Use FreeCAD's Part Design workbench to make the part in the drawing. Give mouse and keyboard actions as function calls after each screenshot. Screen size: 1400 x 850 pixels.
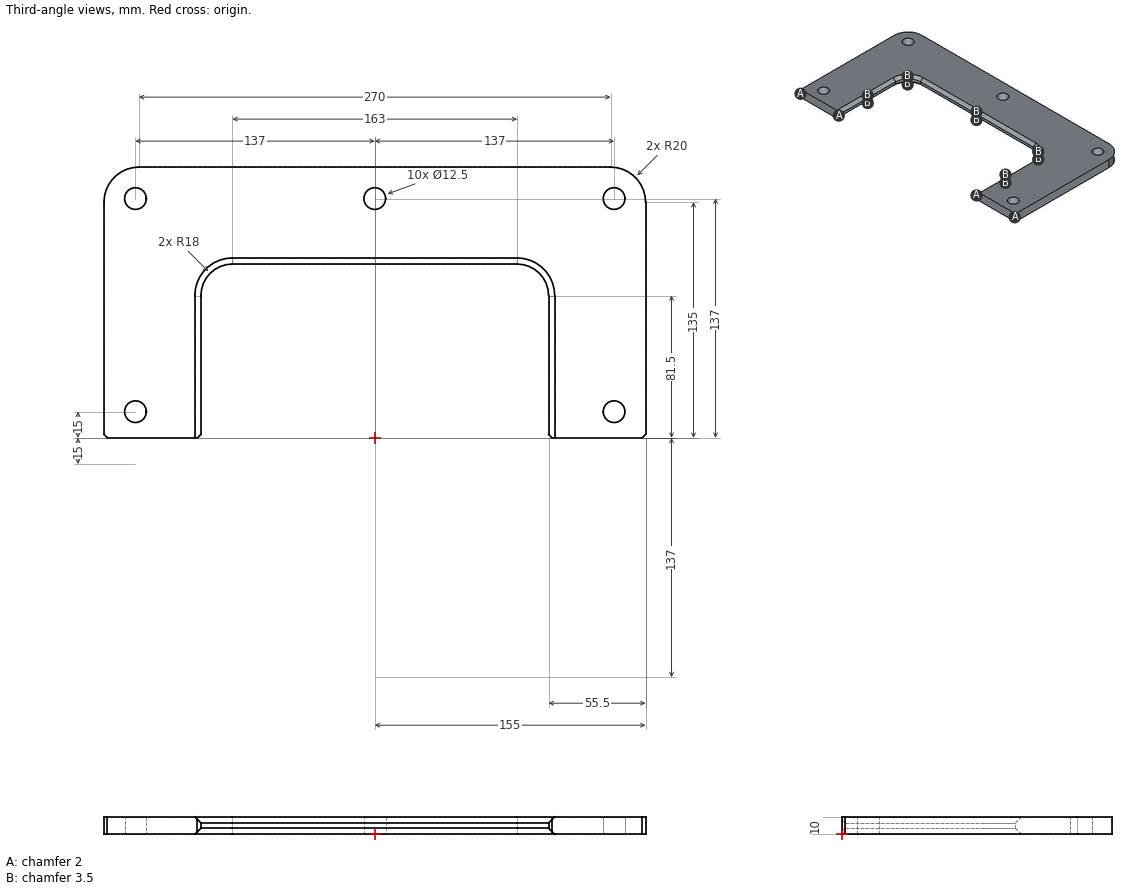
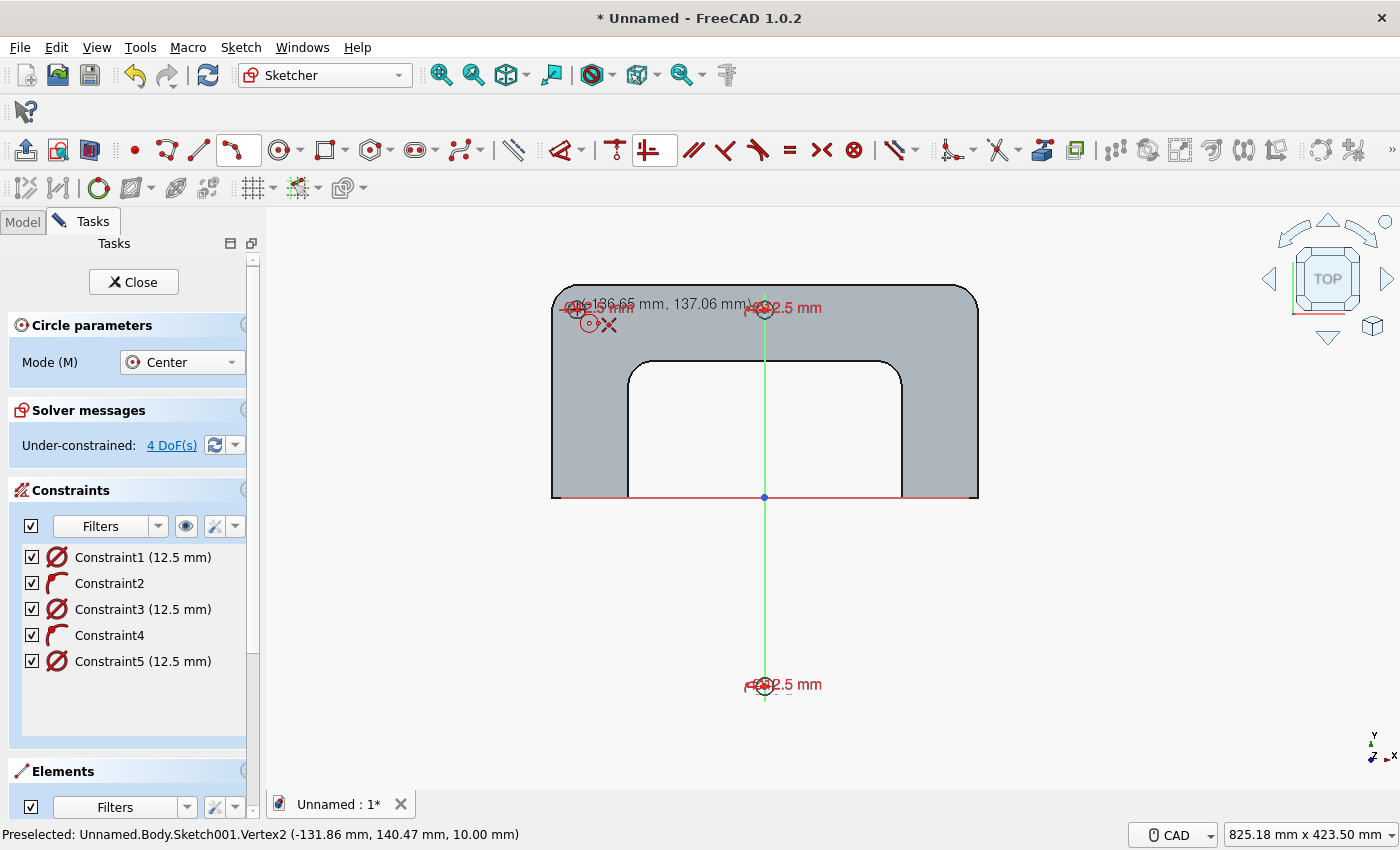
scroll(953, 310, up, 5)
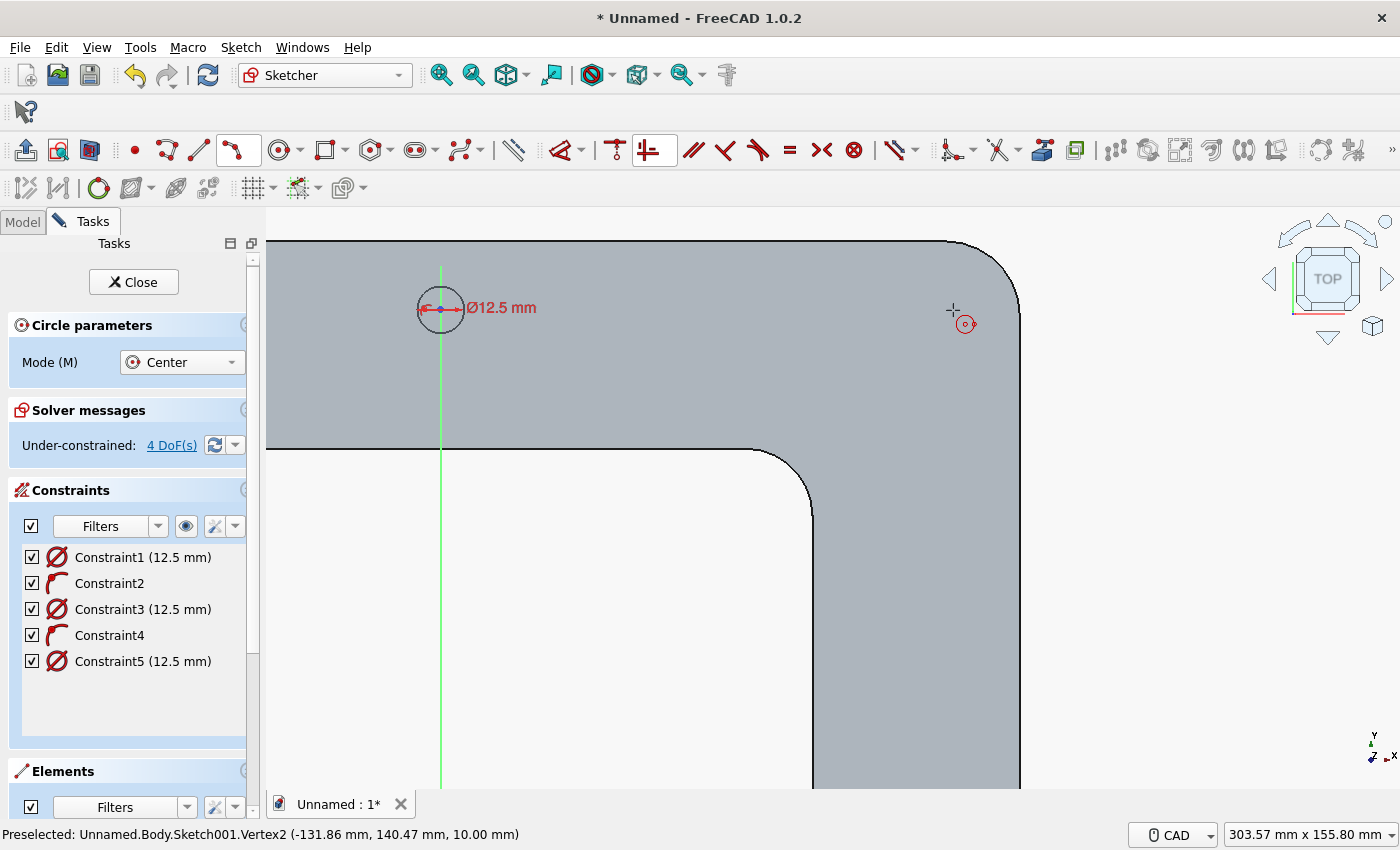
click(953, 309)
move(969, 292)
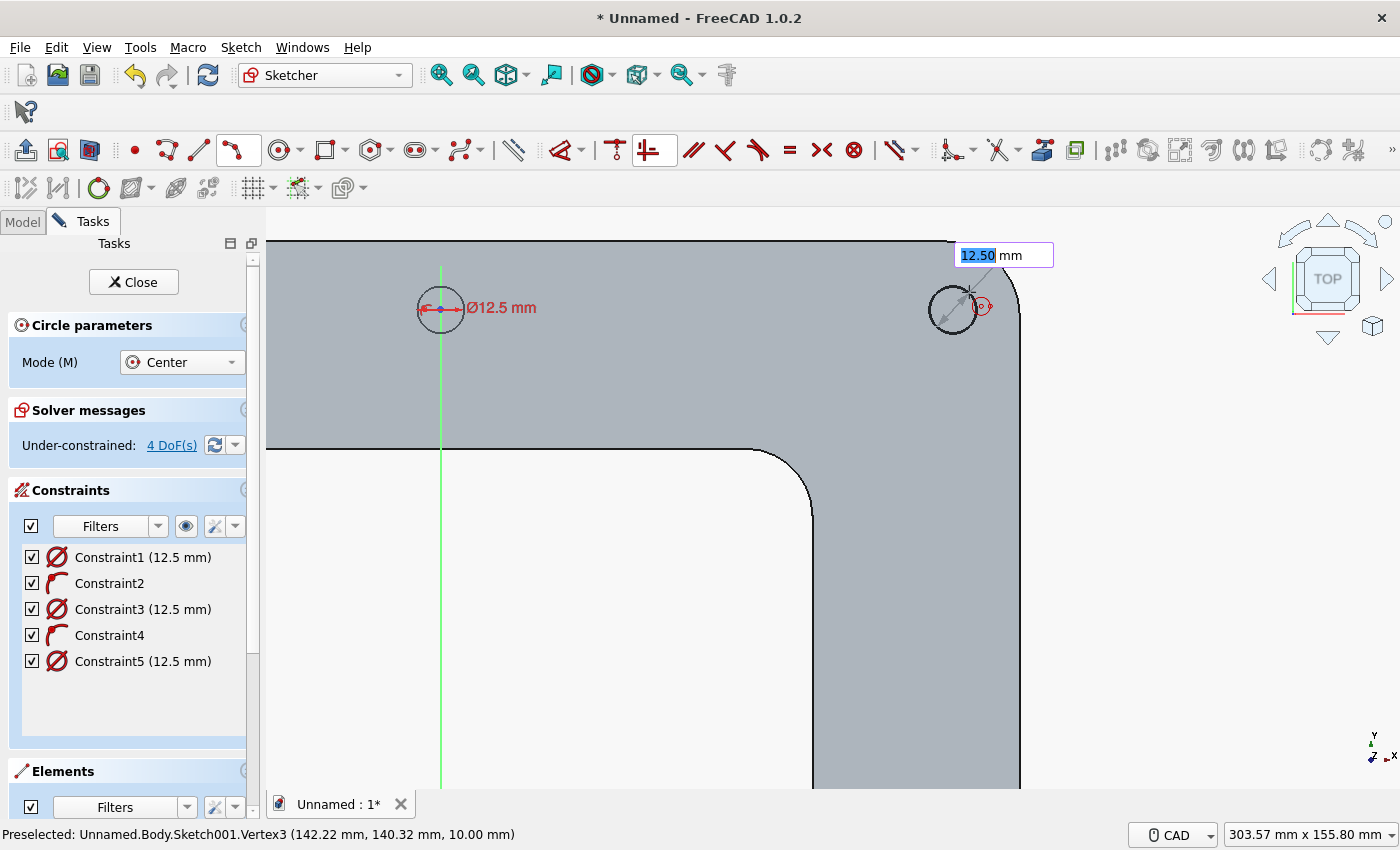
text(12.5)
key(Return)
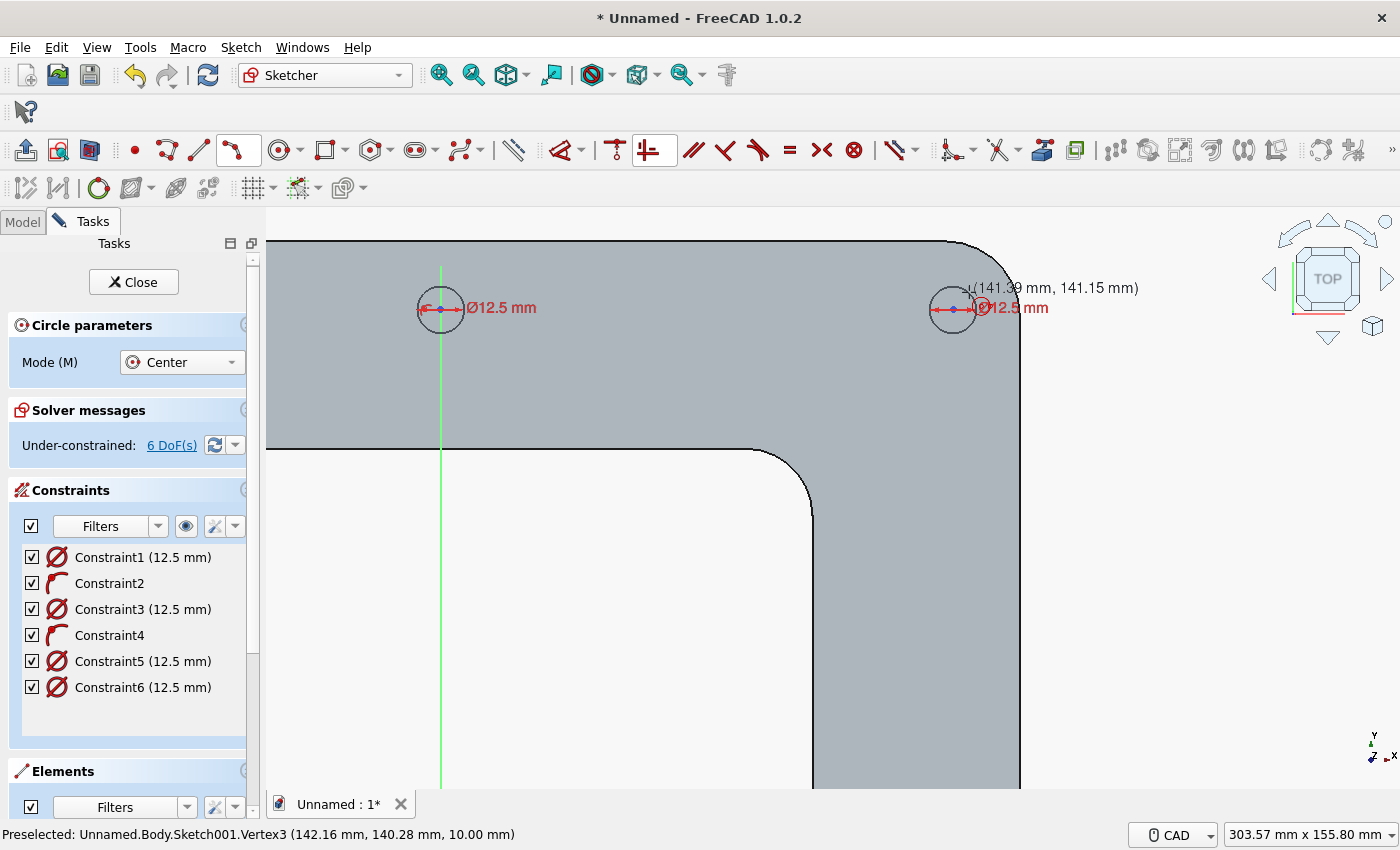
scroll(953, 310, down, 5)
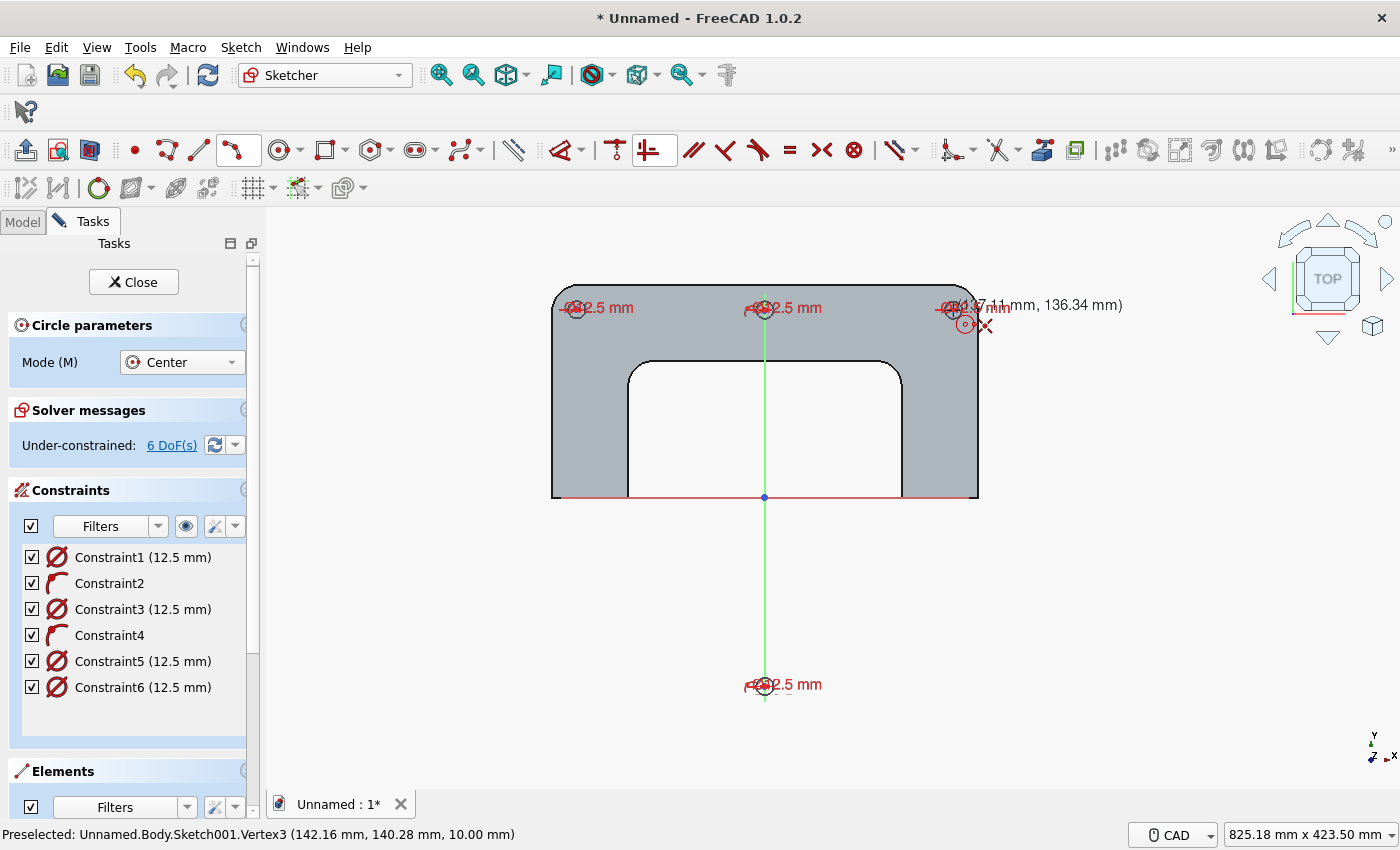
scroll(577, 686, up, 5)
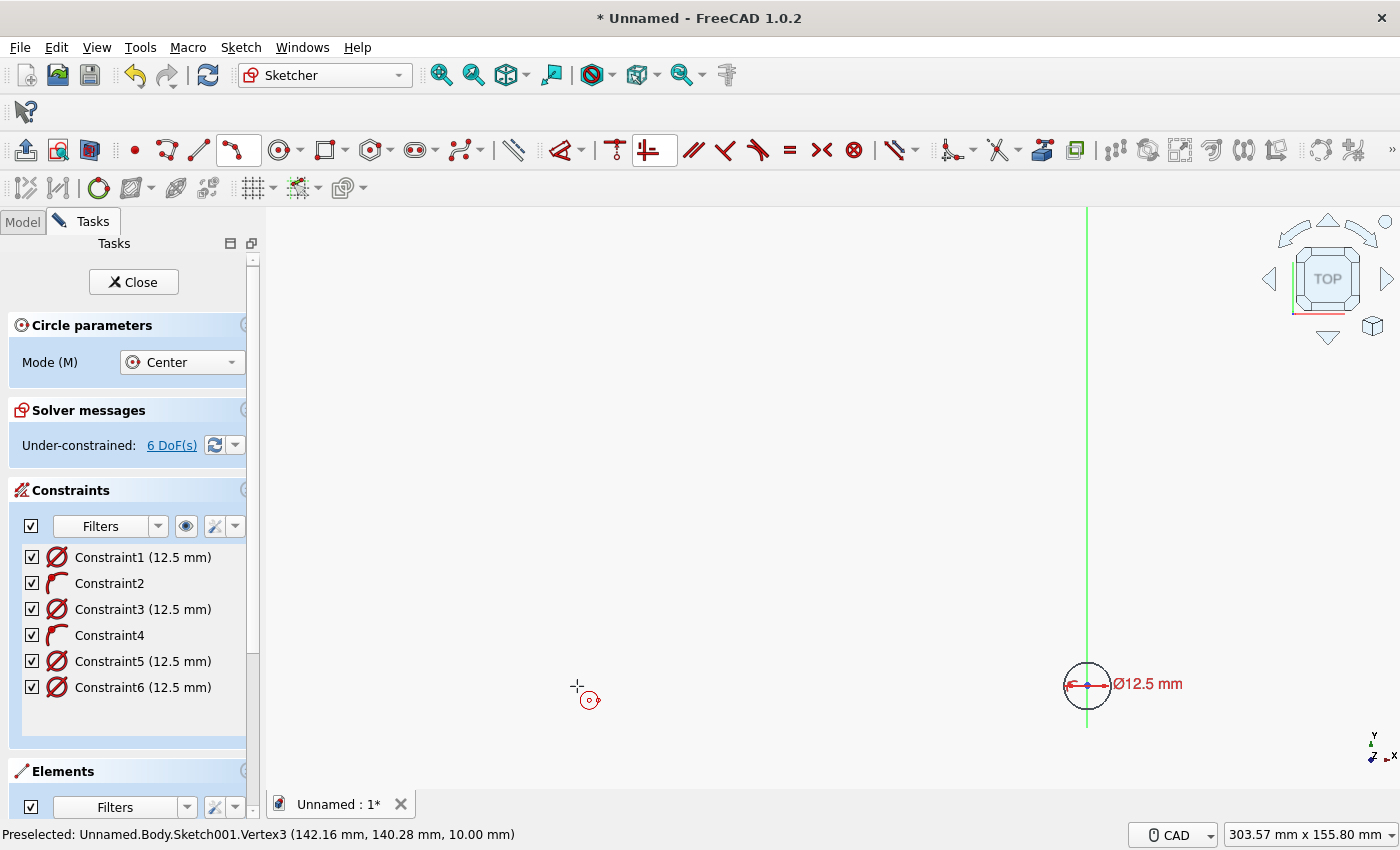
click(576, 685)
move(592, 668)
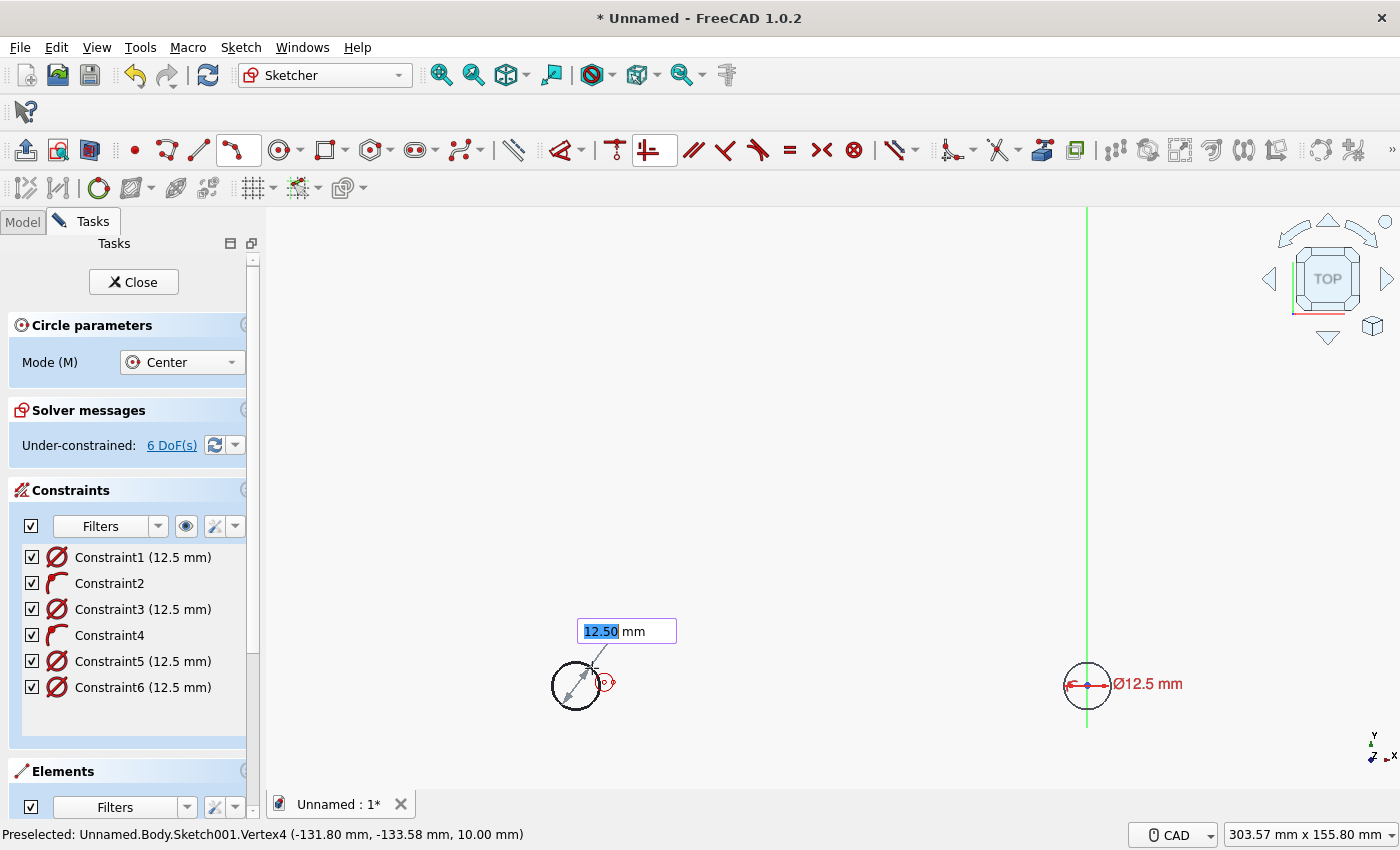
text(12.5)
key(Return)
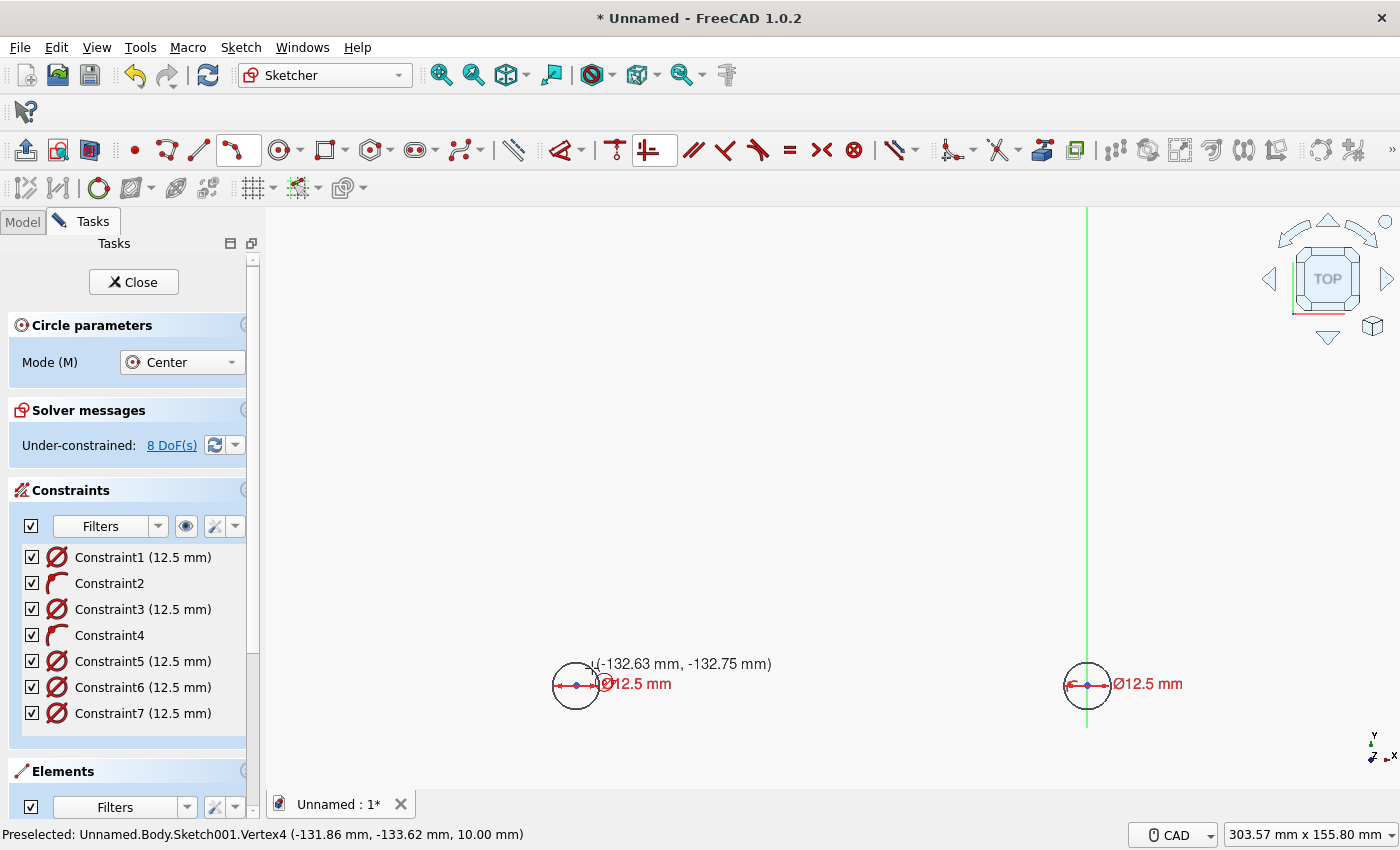
scroll(577, 687, down, 5)